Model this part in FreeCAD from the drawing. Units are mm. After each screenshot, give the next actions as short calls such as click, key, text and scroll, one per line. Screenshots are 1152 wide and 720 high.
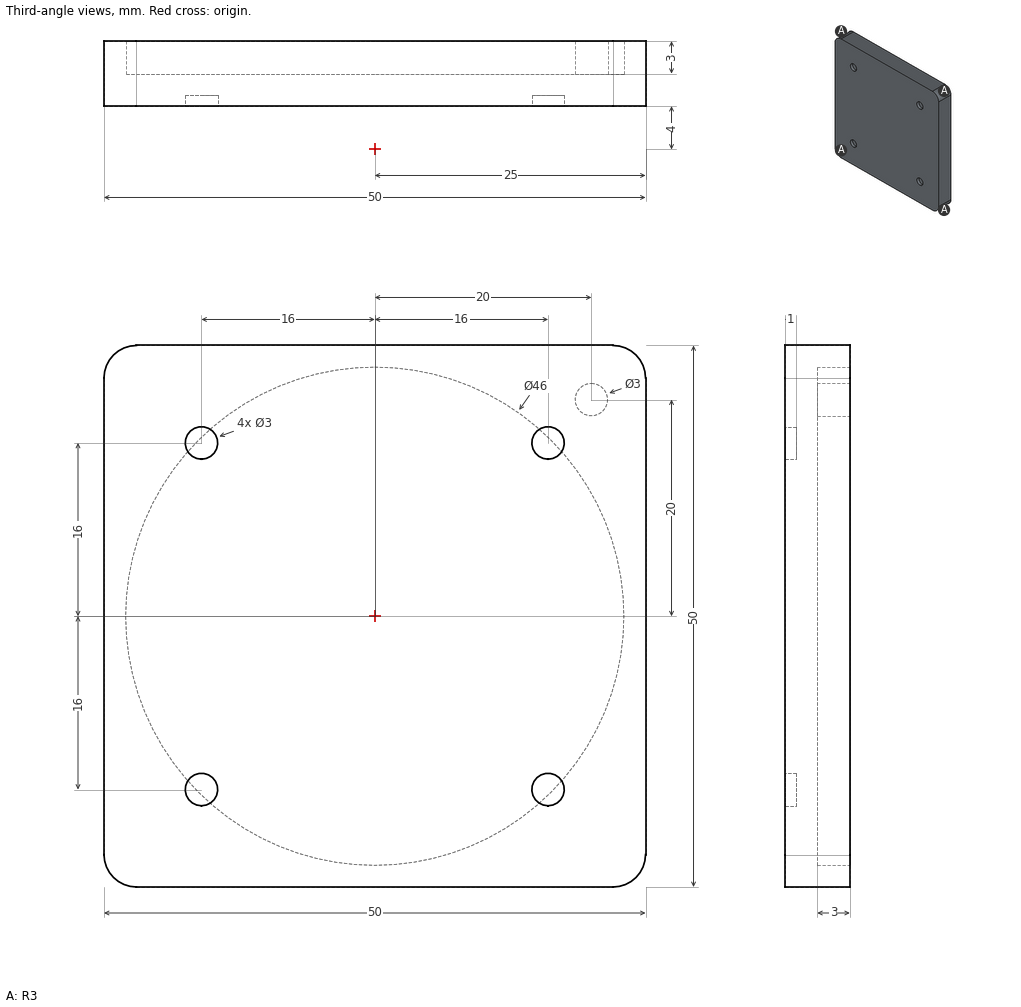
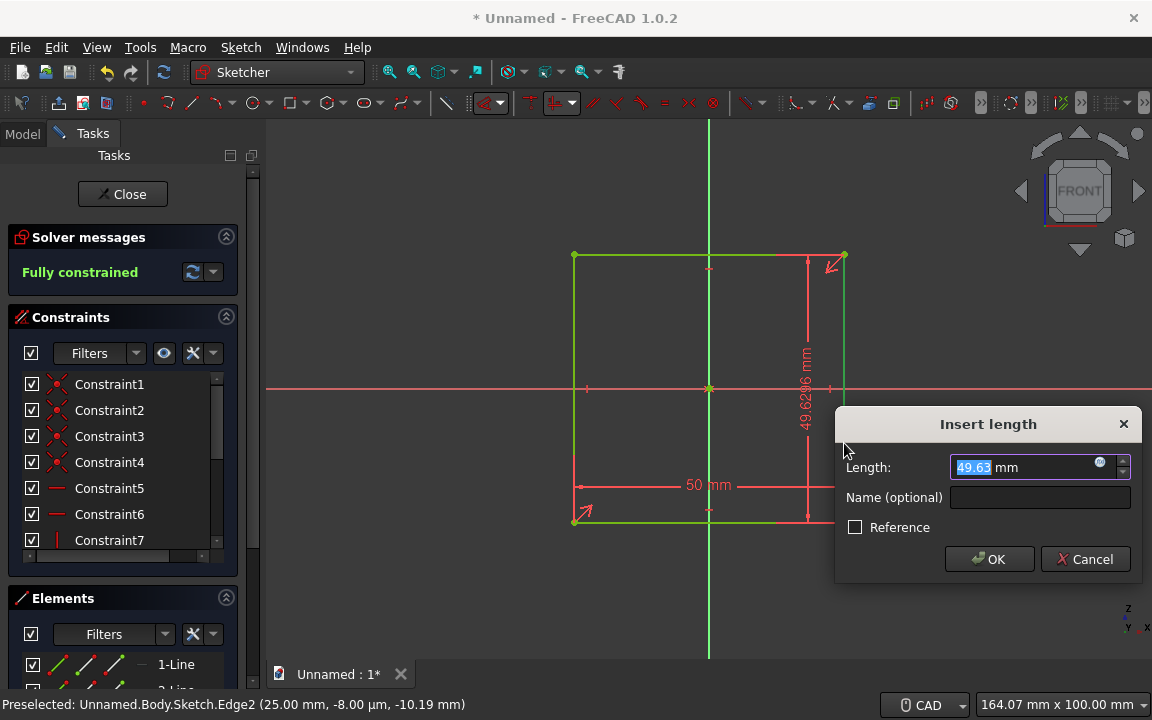
text(50)
key(Return)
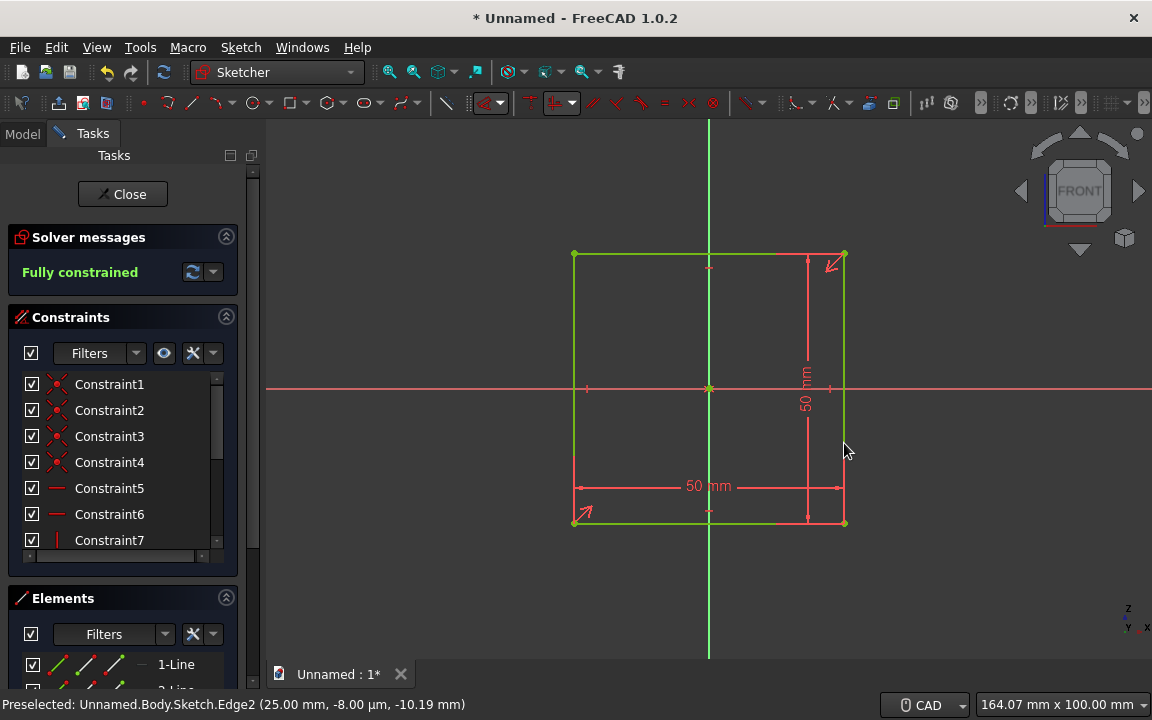
click(123, 194)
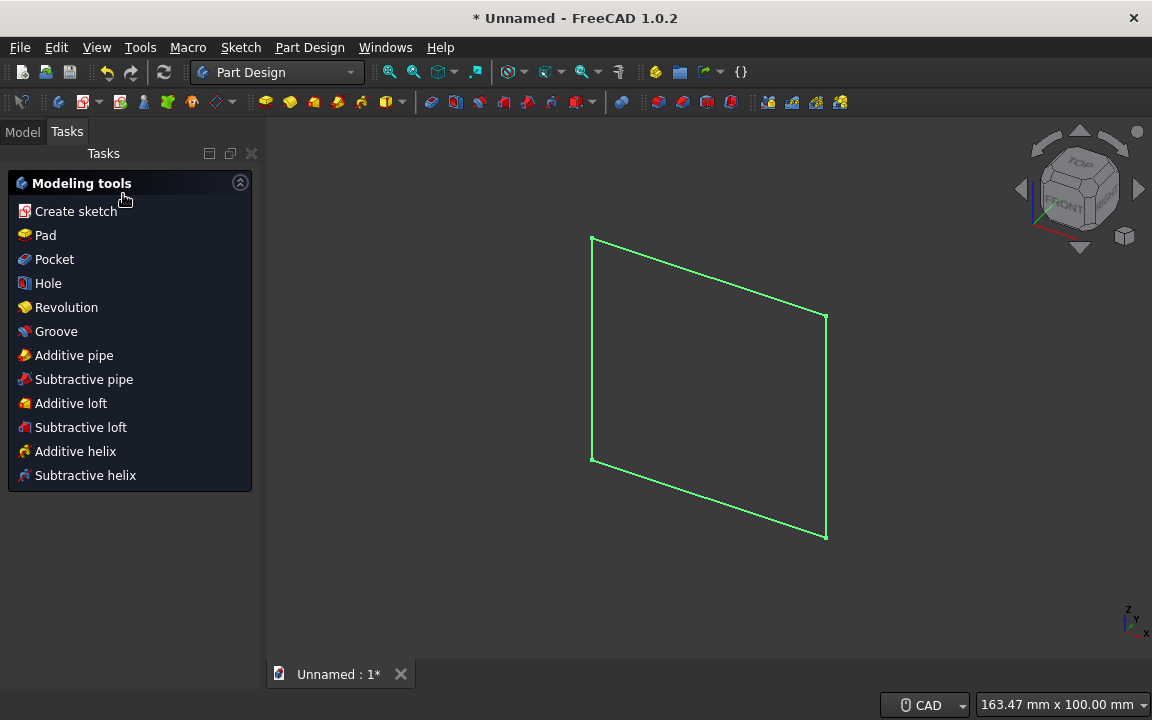
click(266, 102)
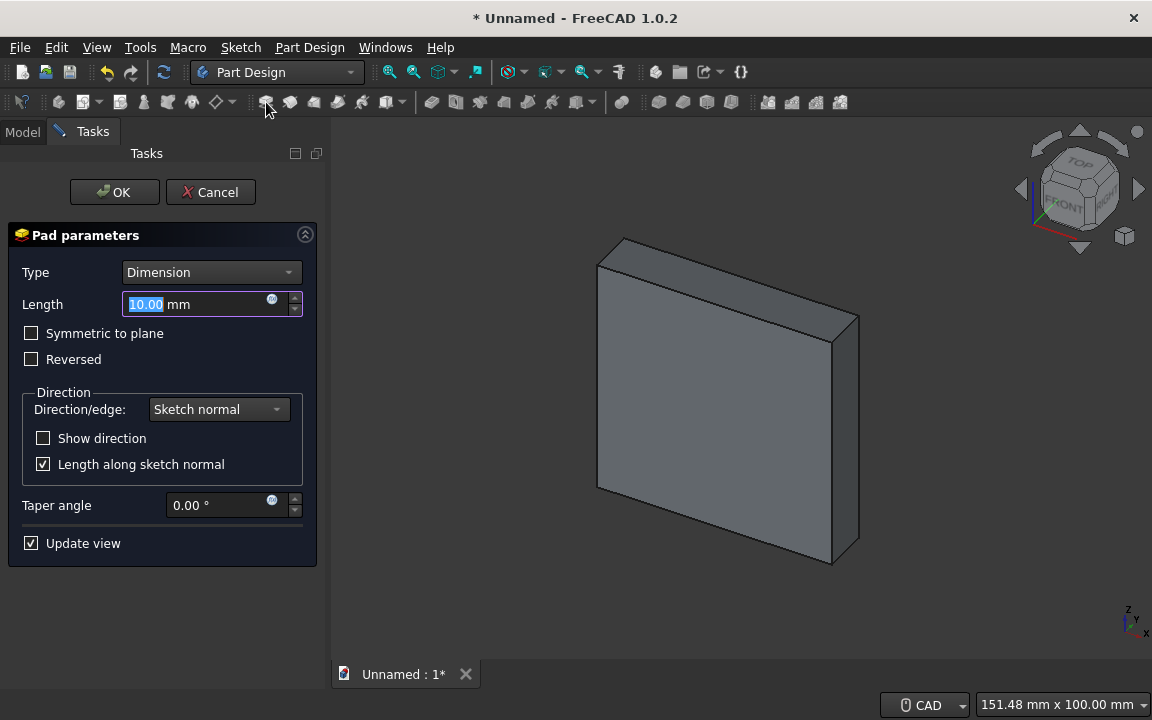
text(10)
key(Tab)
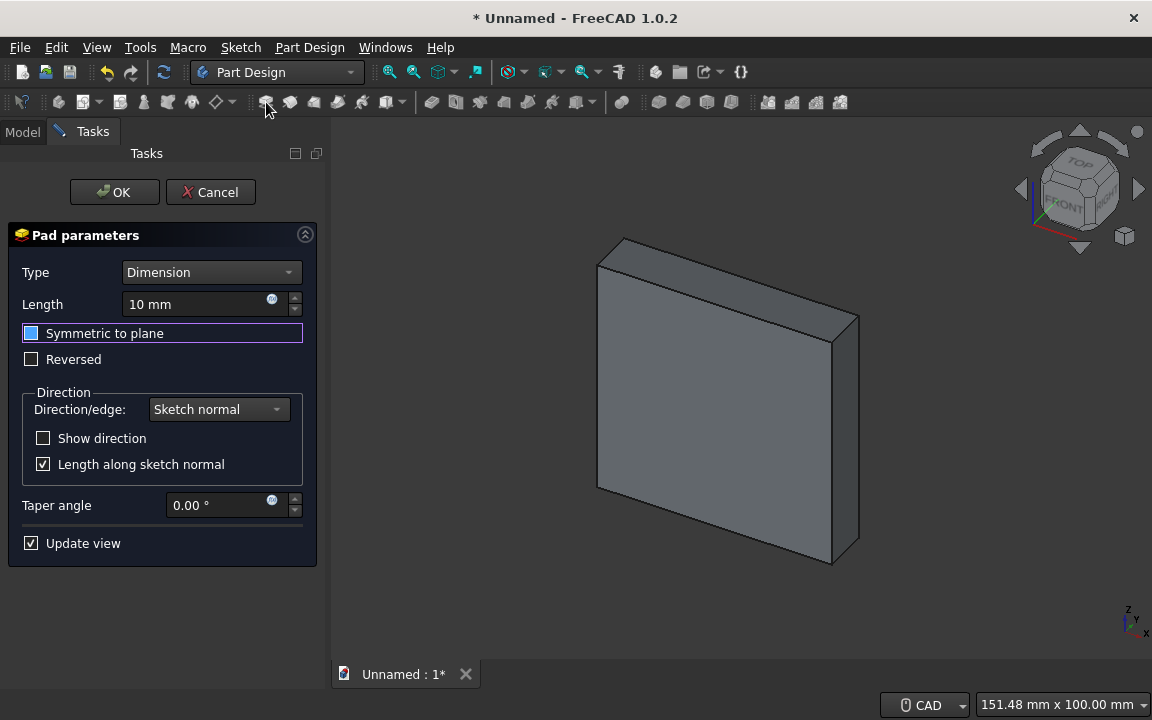
click(30, 359)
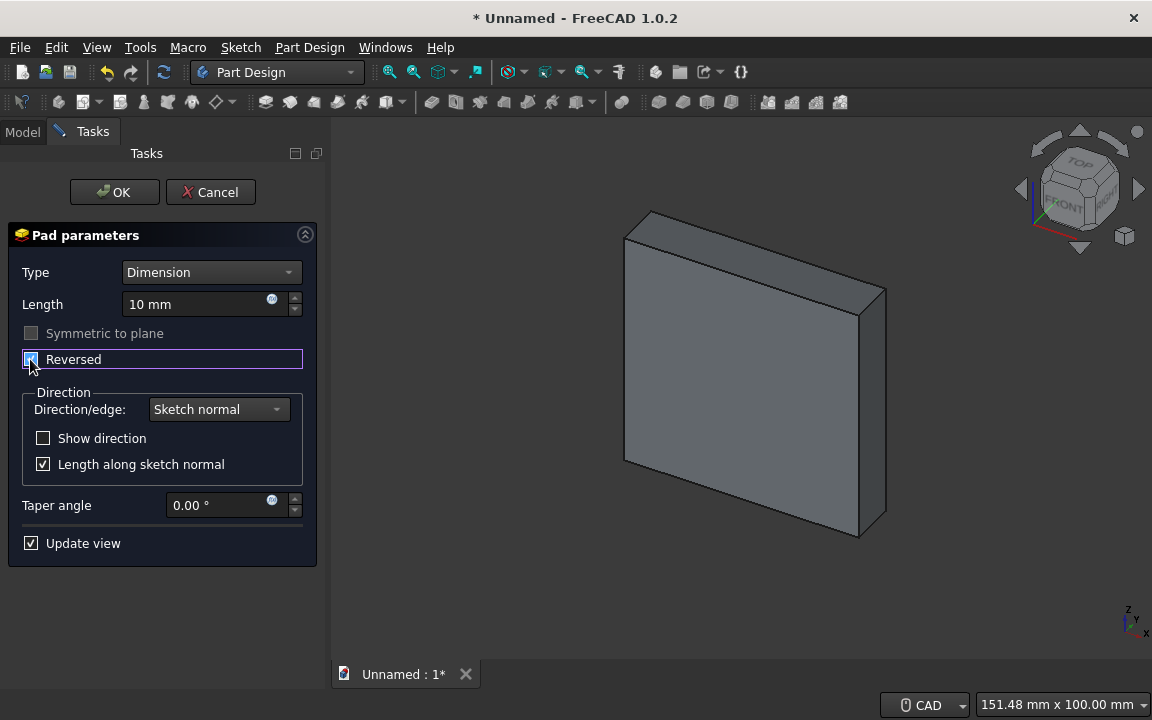
click(115, 192)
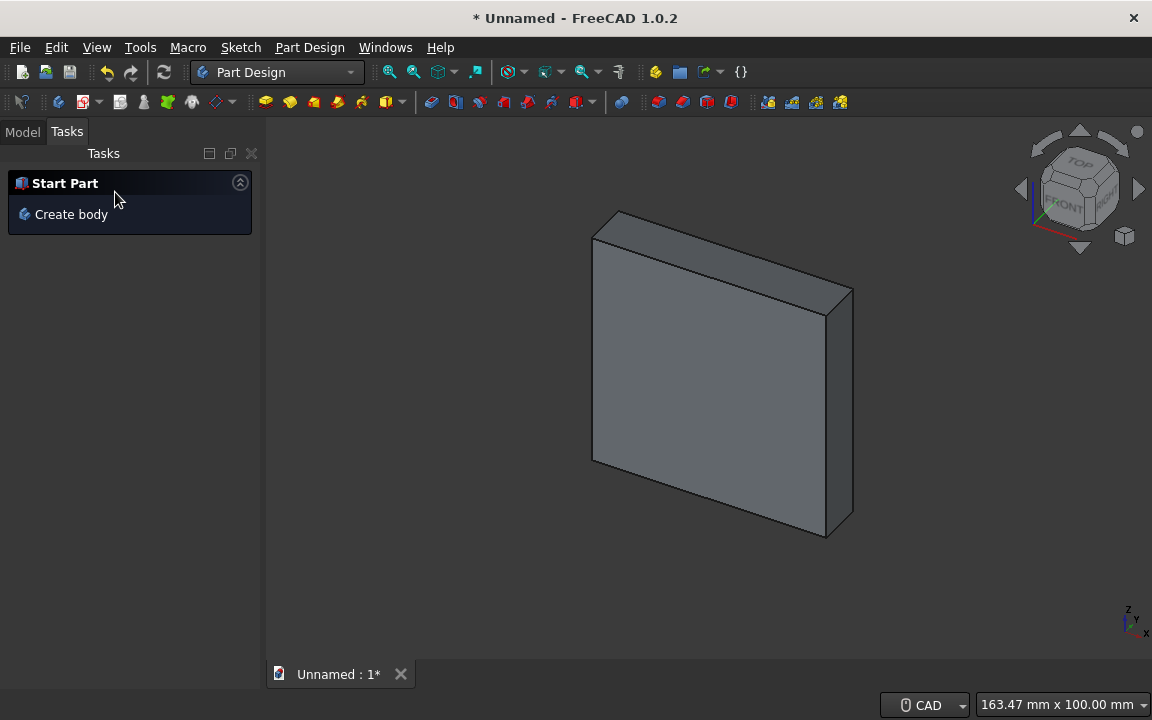
key(4)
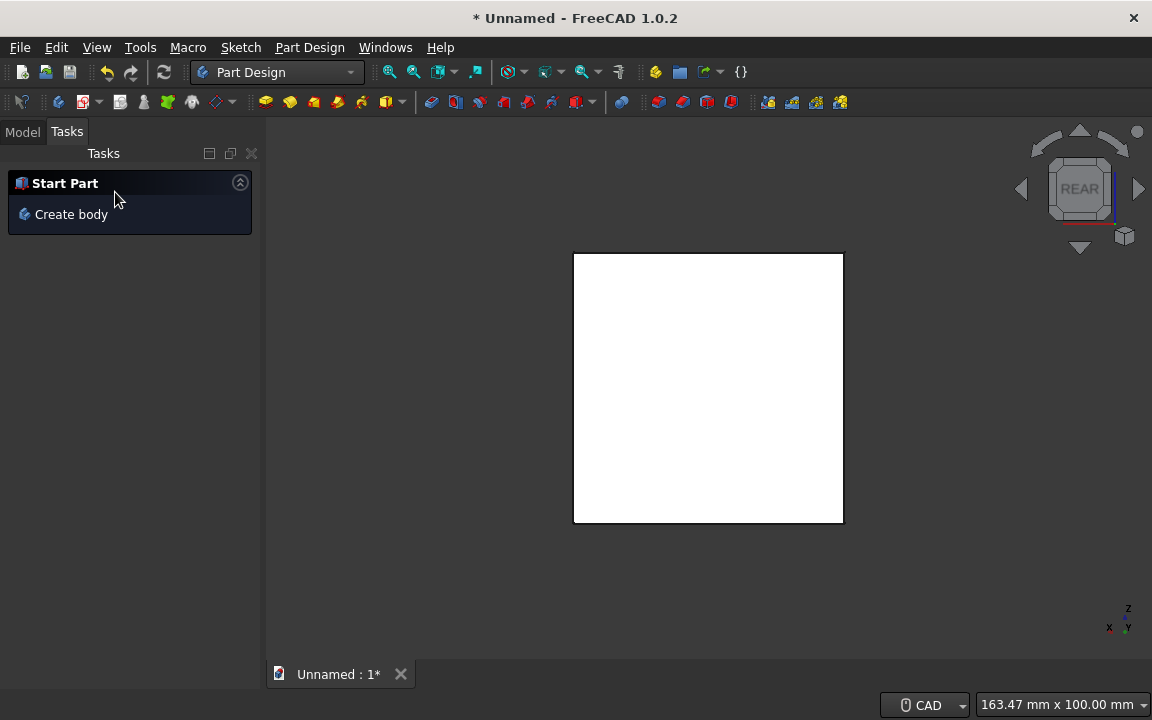
click(709, 387)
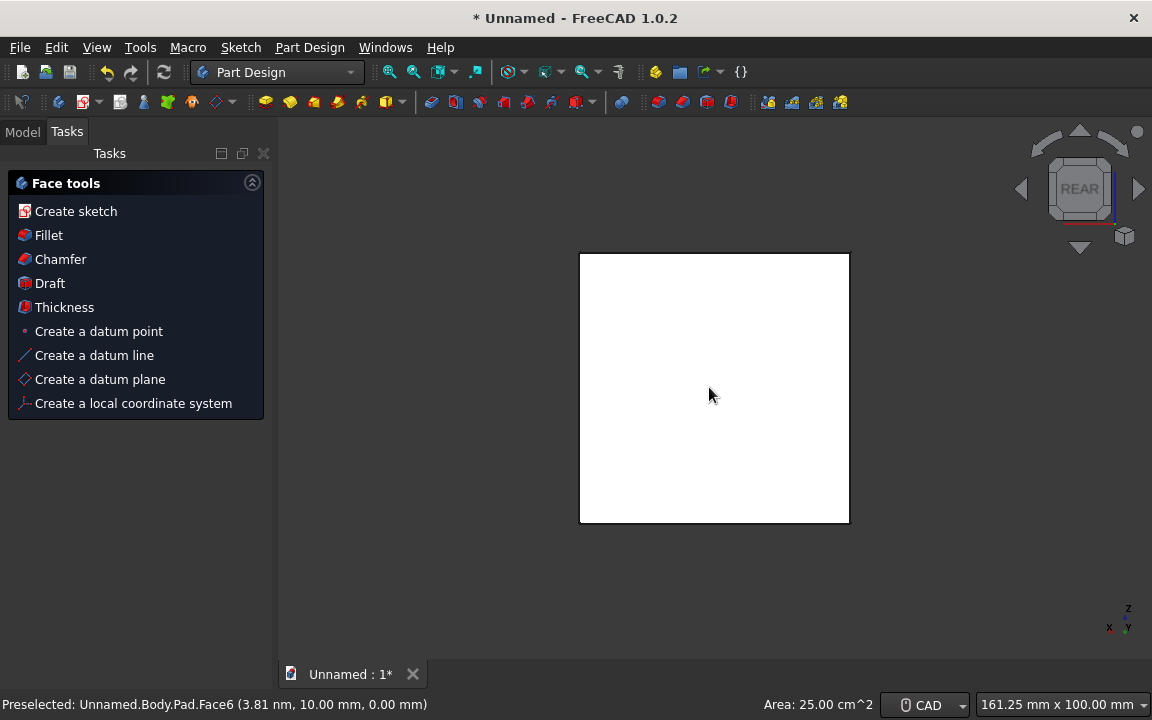
click(84, 102)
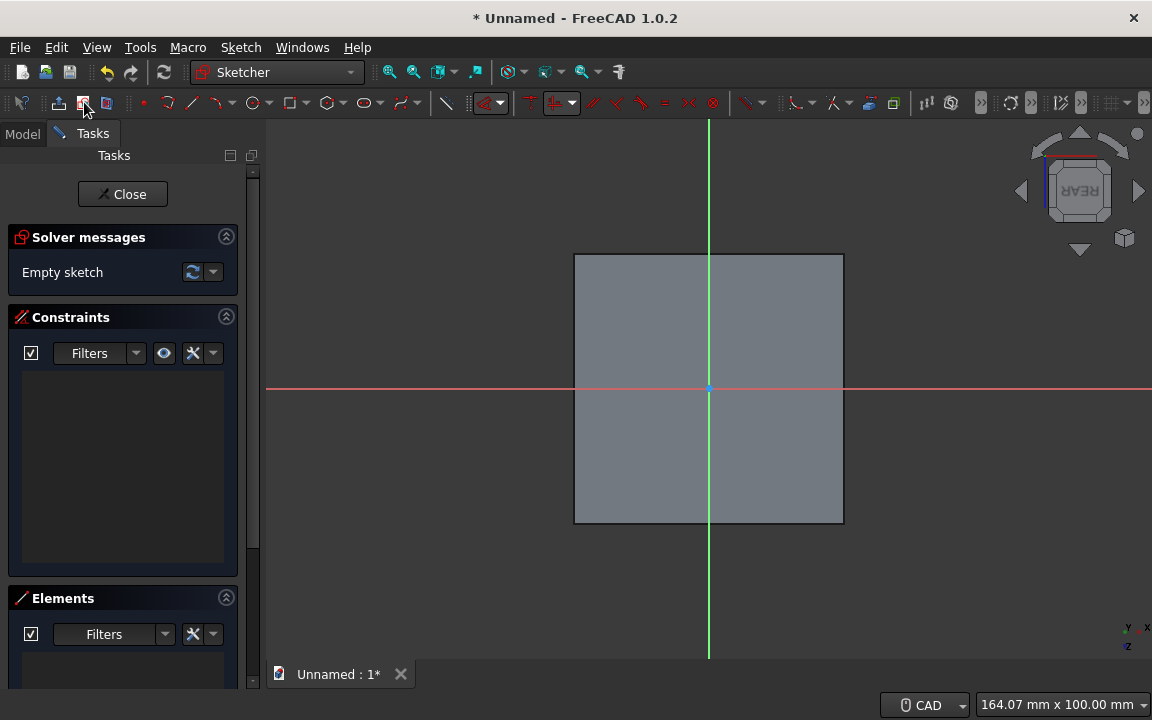
scroll(848, 389, up, 2)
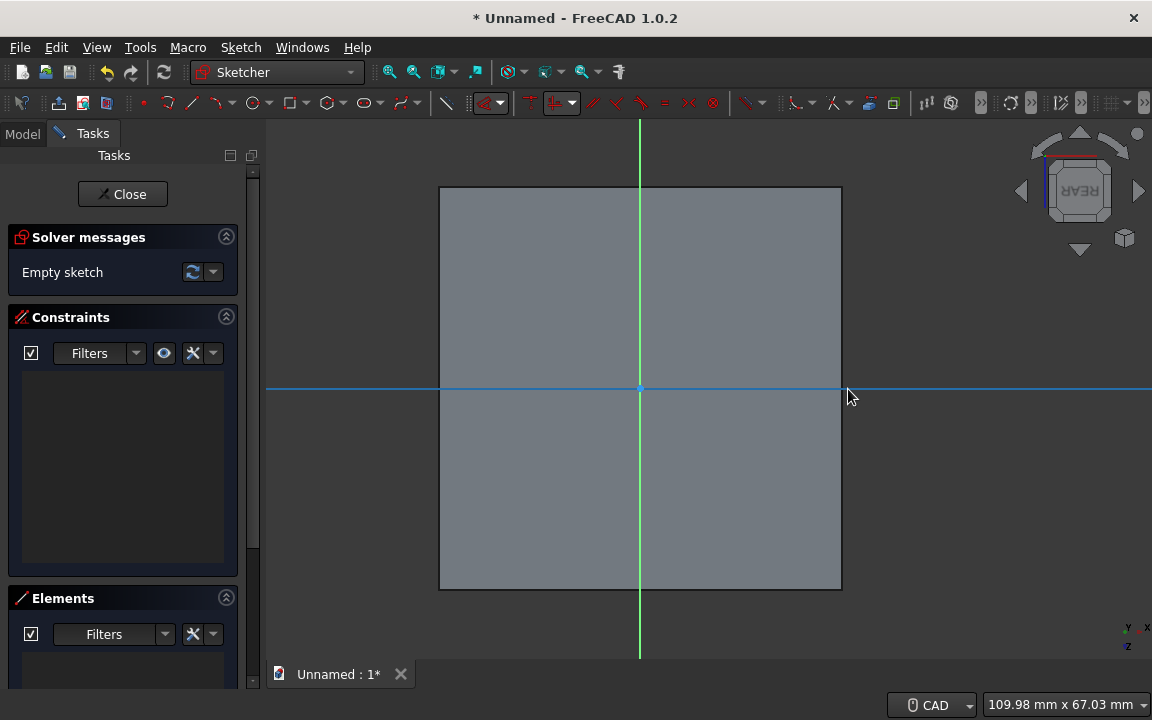
click(254, 104)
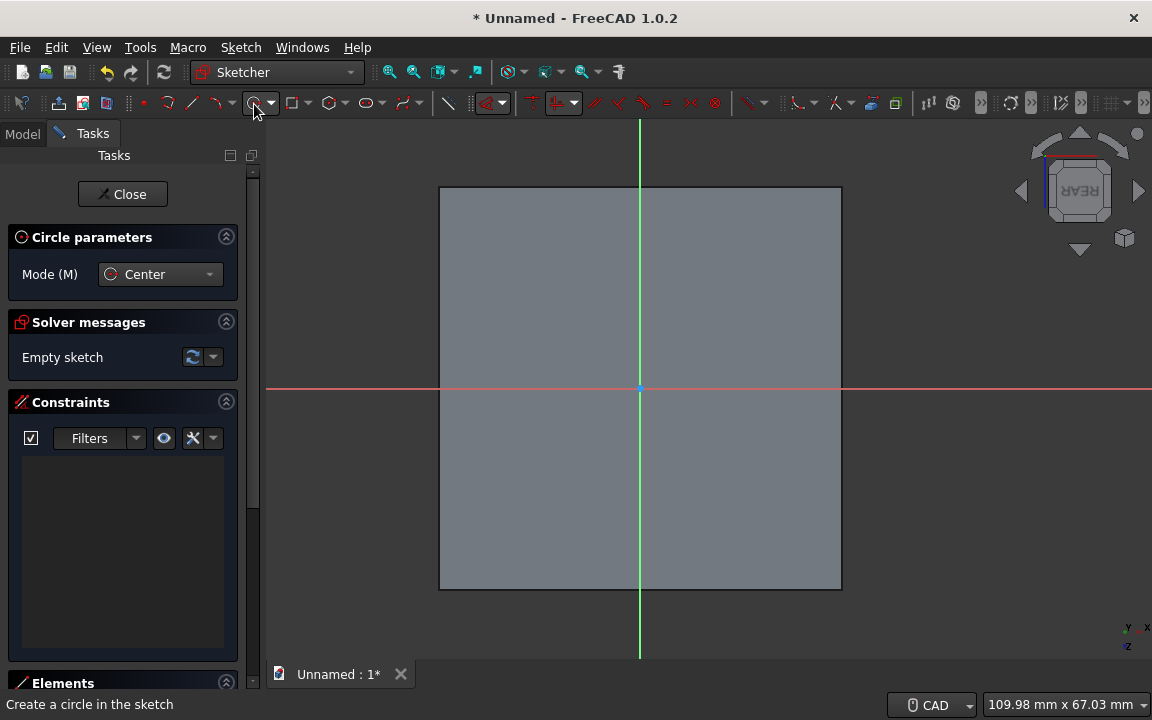
click(640, 389)
click(771, 258)
key(Escape)